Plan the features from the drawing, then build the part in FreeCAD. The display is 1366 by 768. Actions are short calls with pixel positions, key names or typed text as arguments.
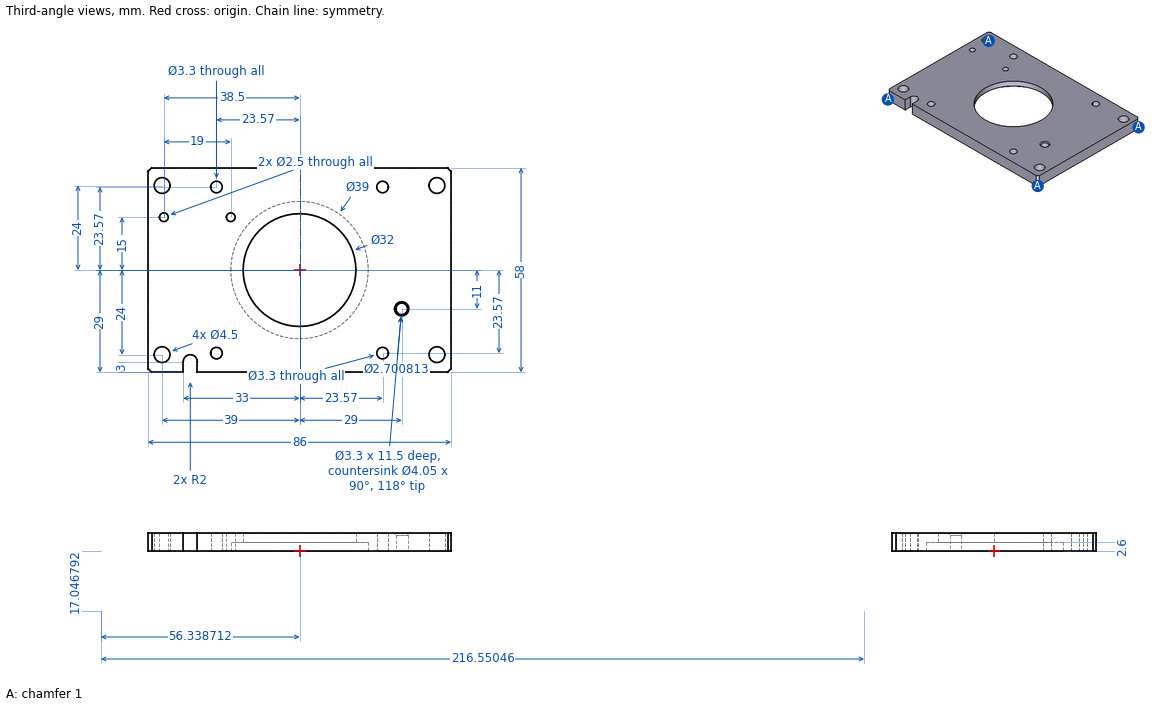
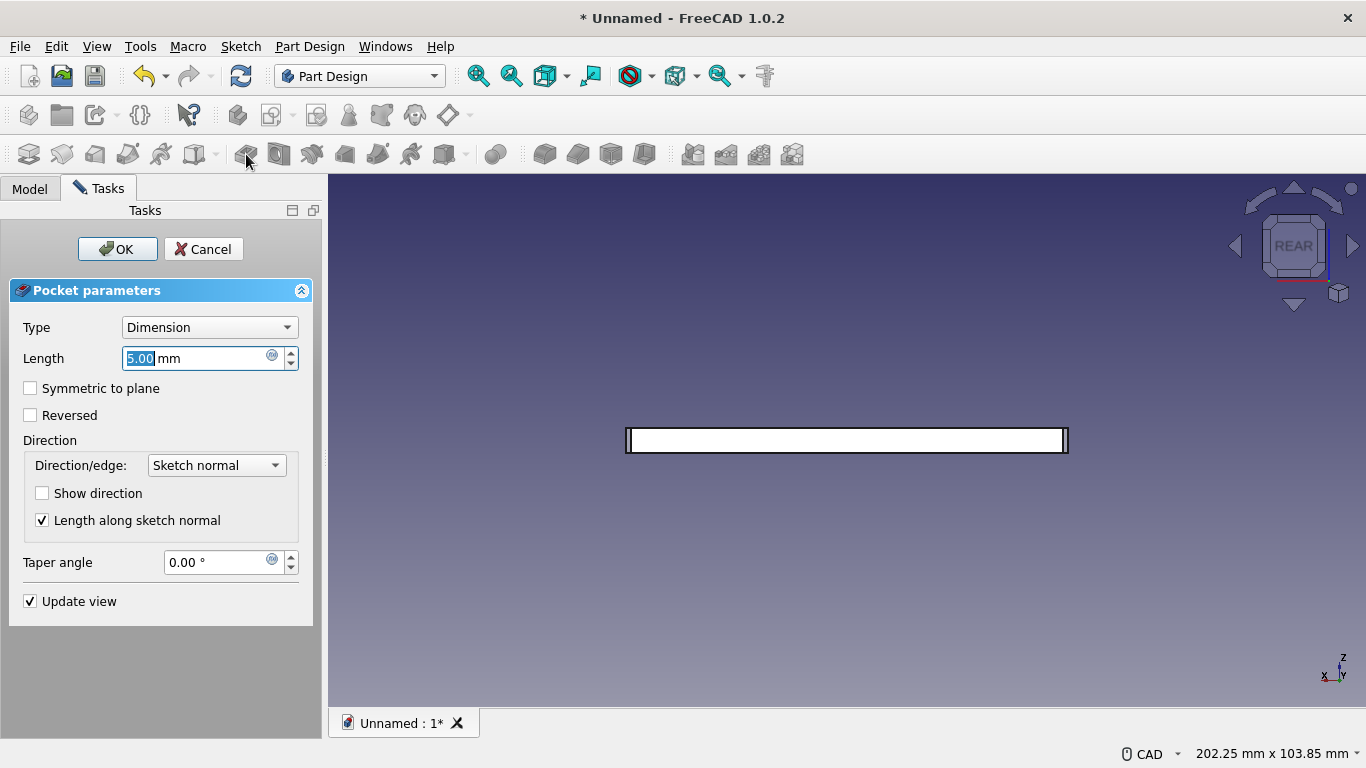
text(2.6)
key(Tab)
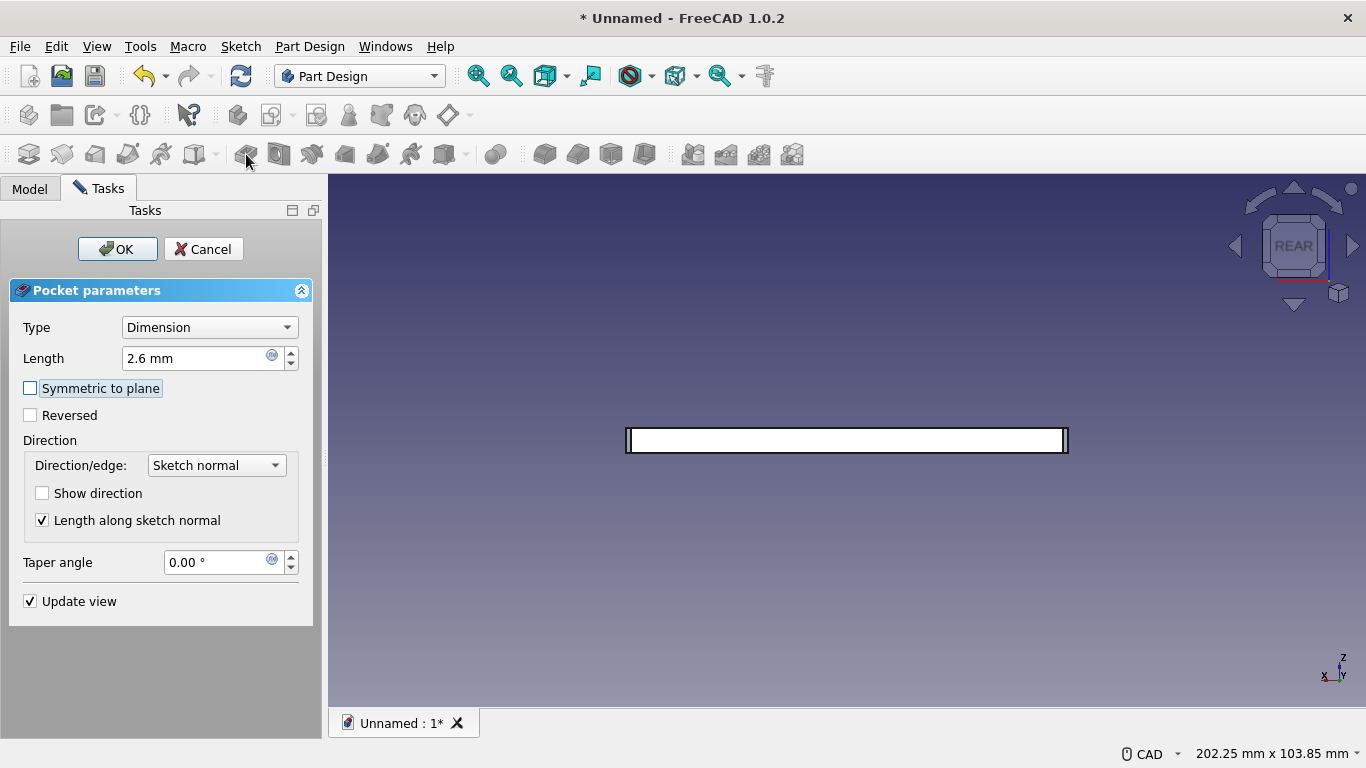
click(31, 415)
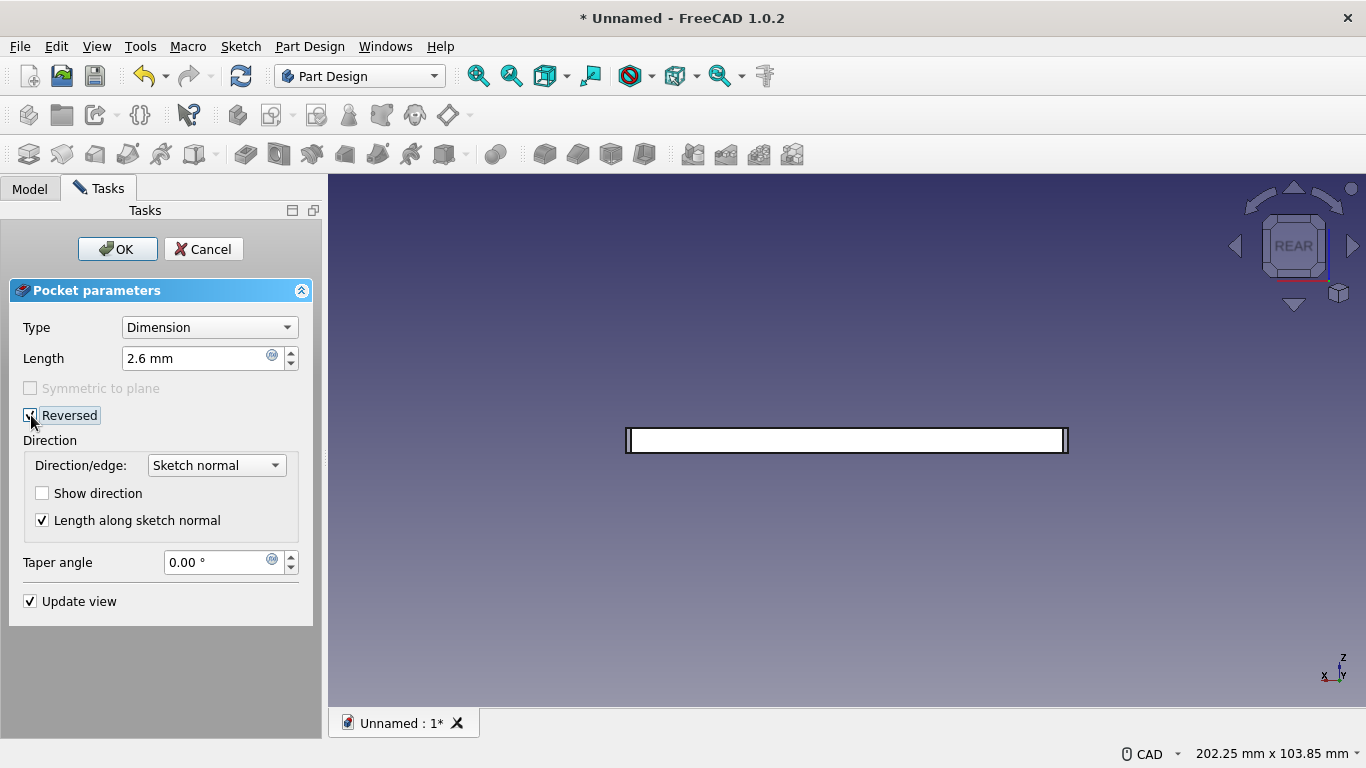
click(118, 249)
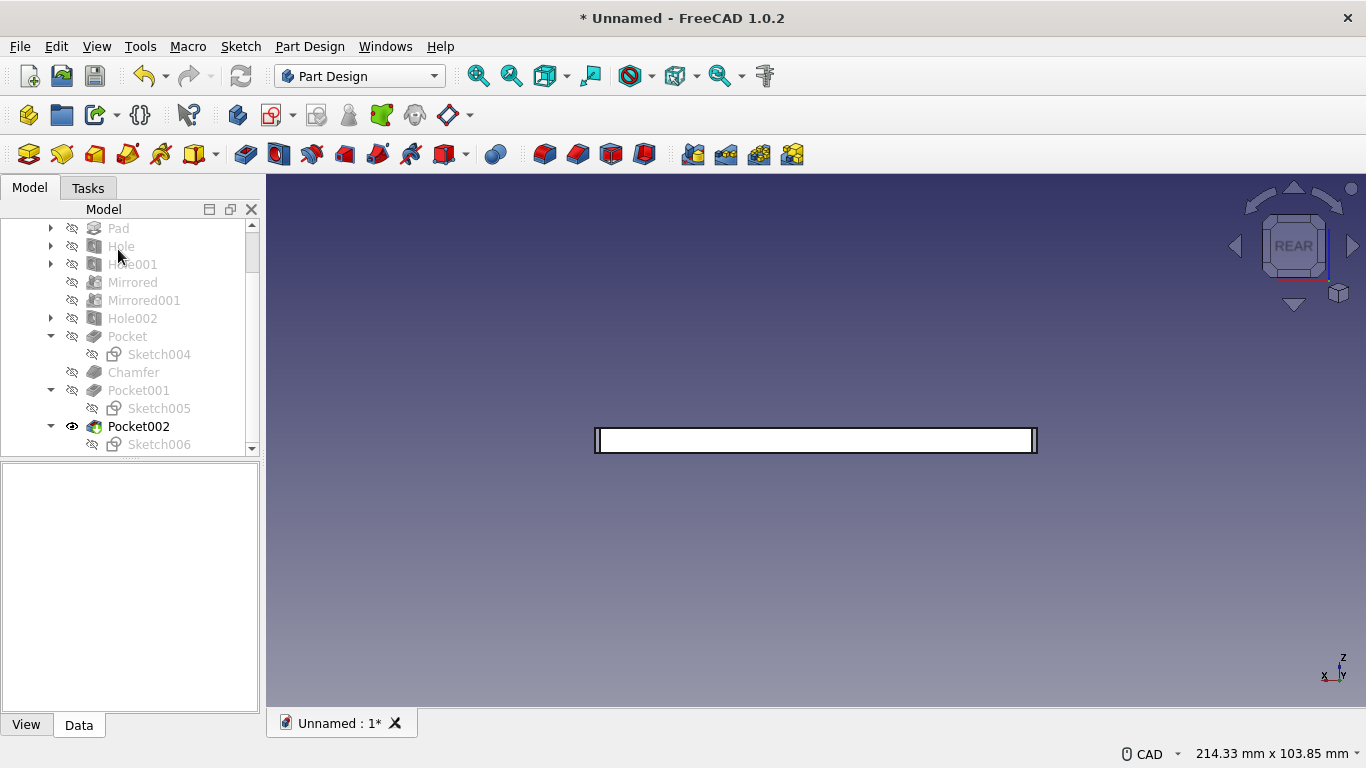
click(479, 76)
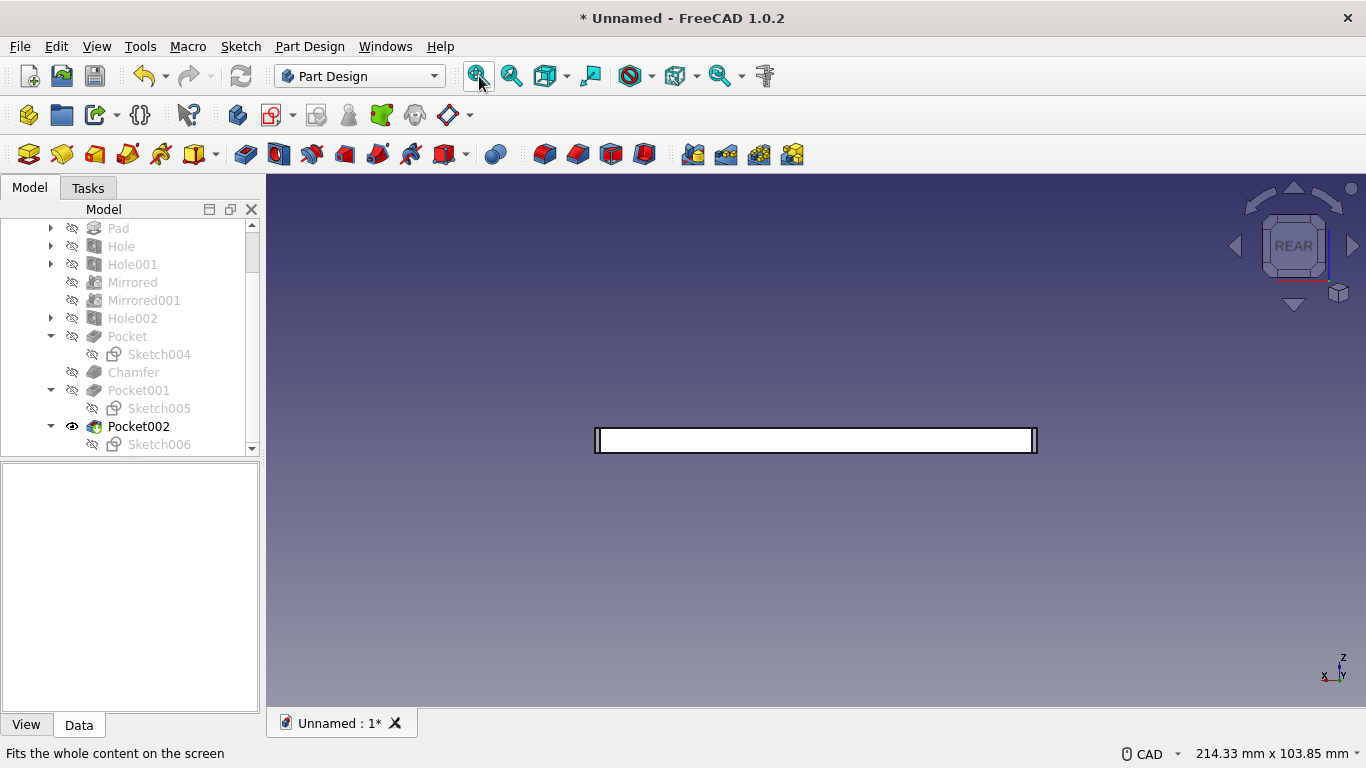
key(0)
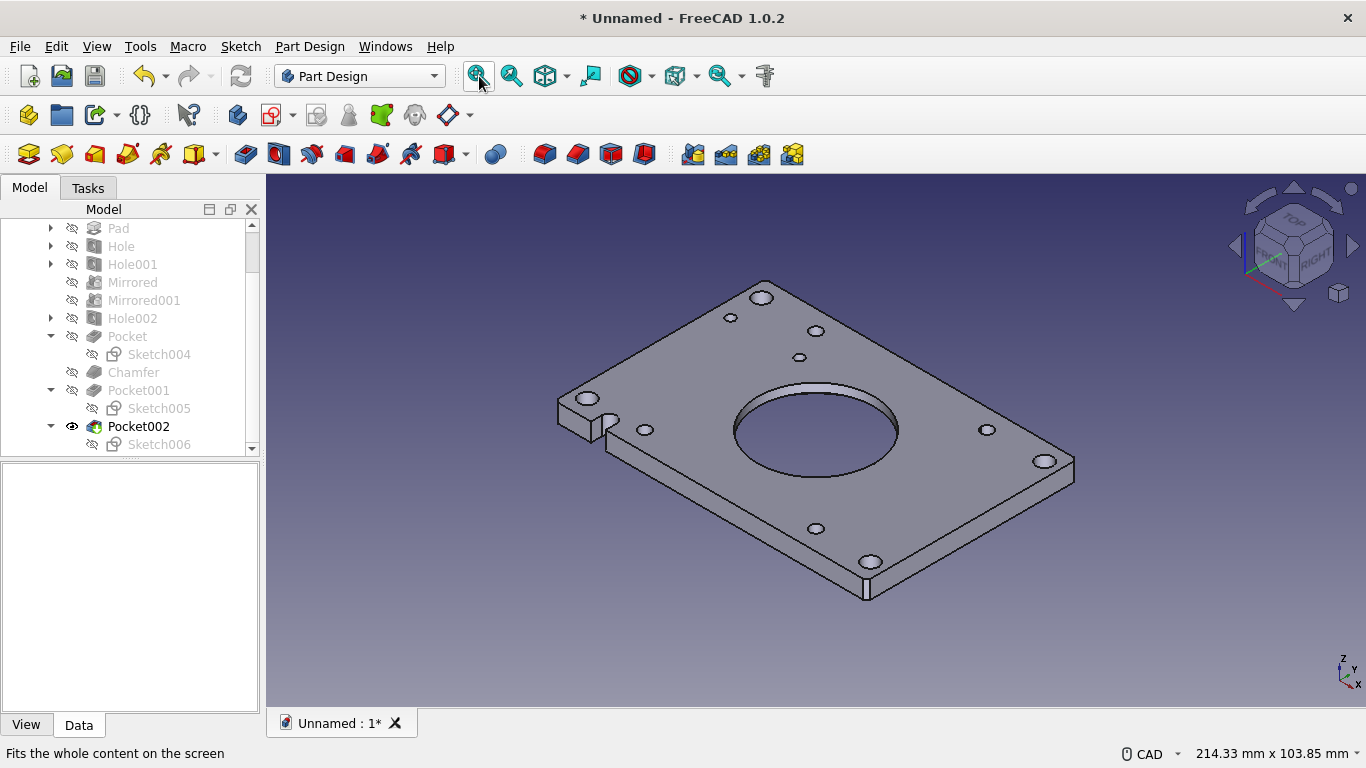
click(697, 395)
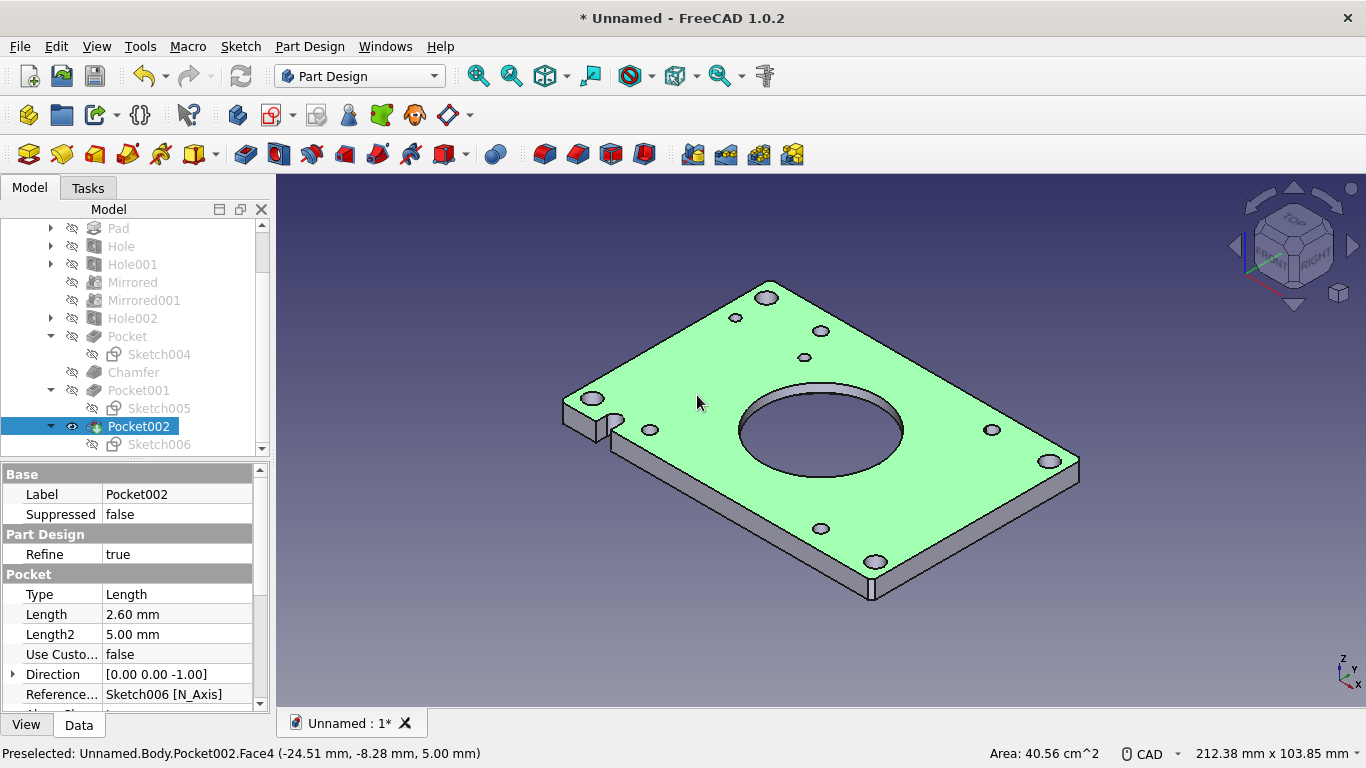
click(270, 116)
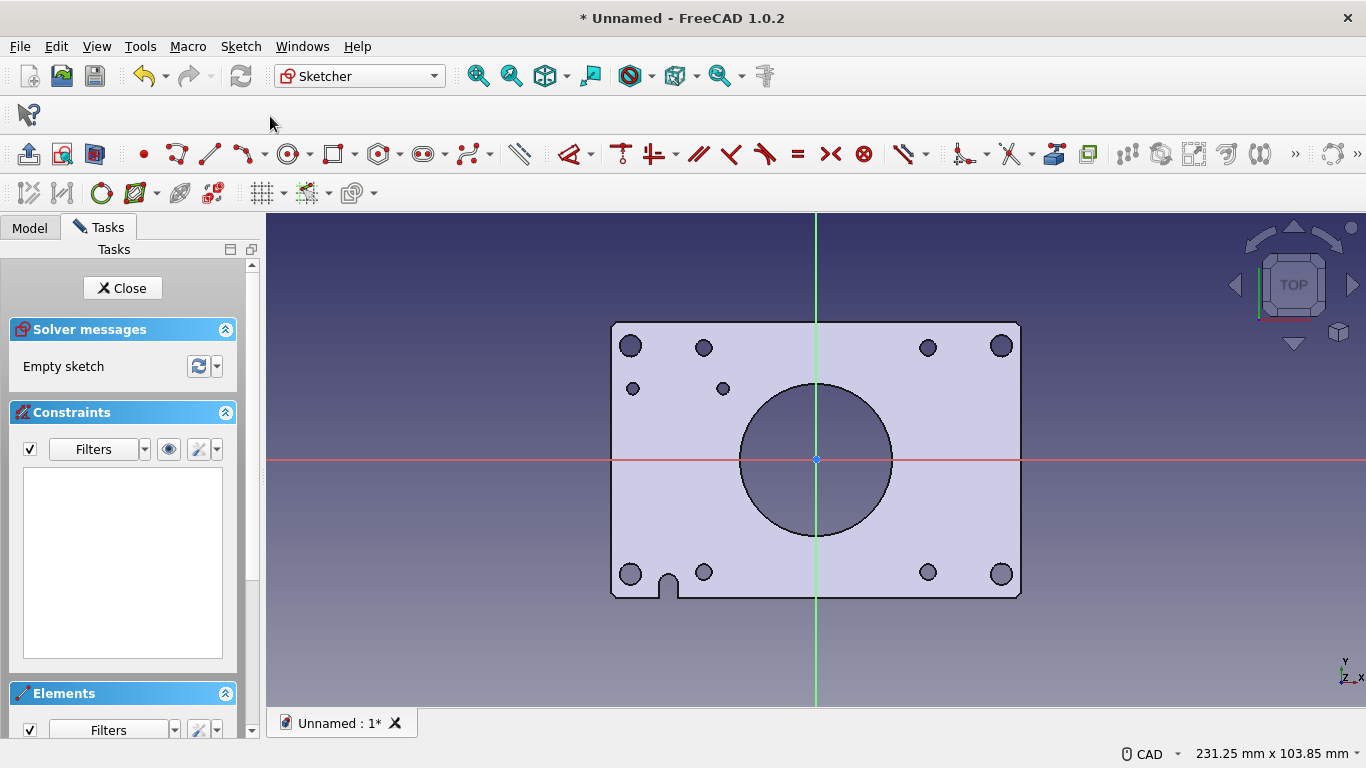
scroll(965, 515, up, 15)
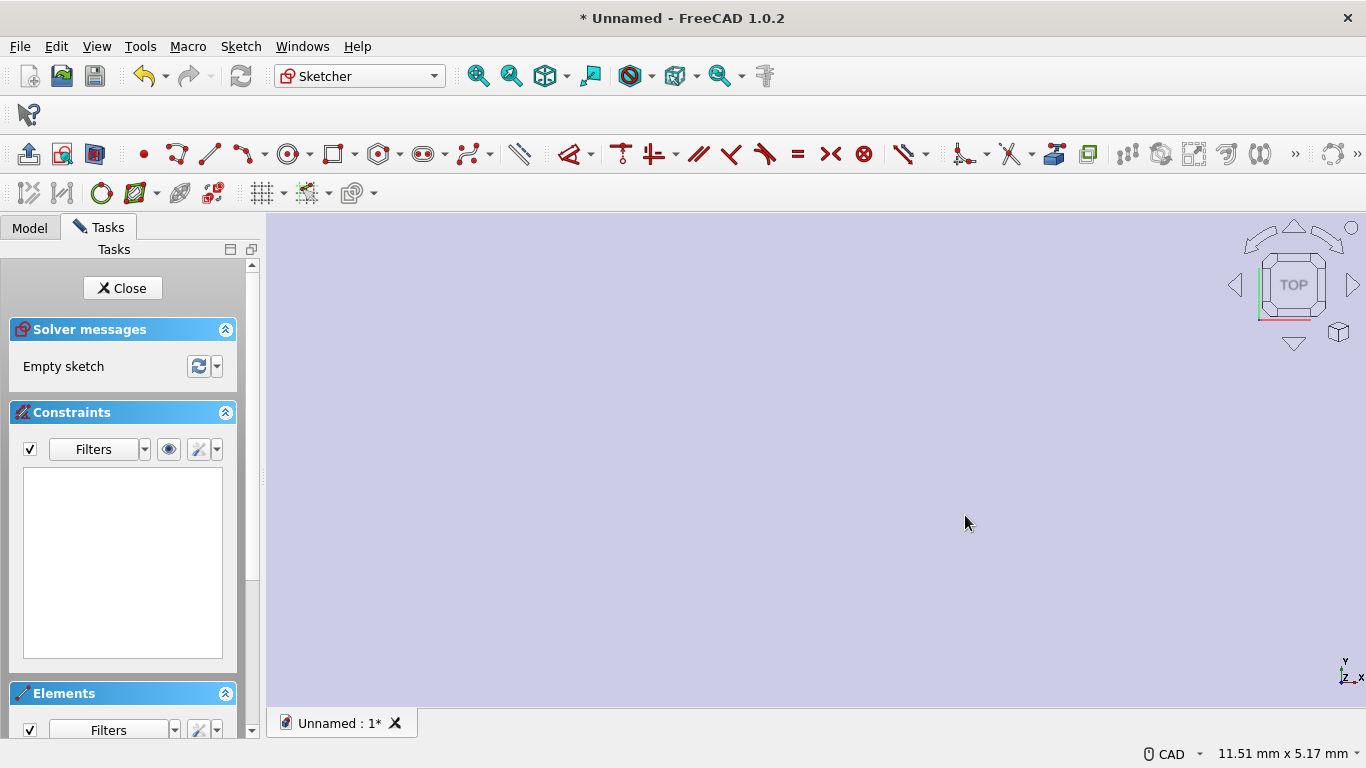
click(288, 154)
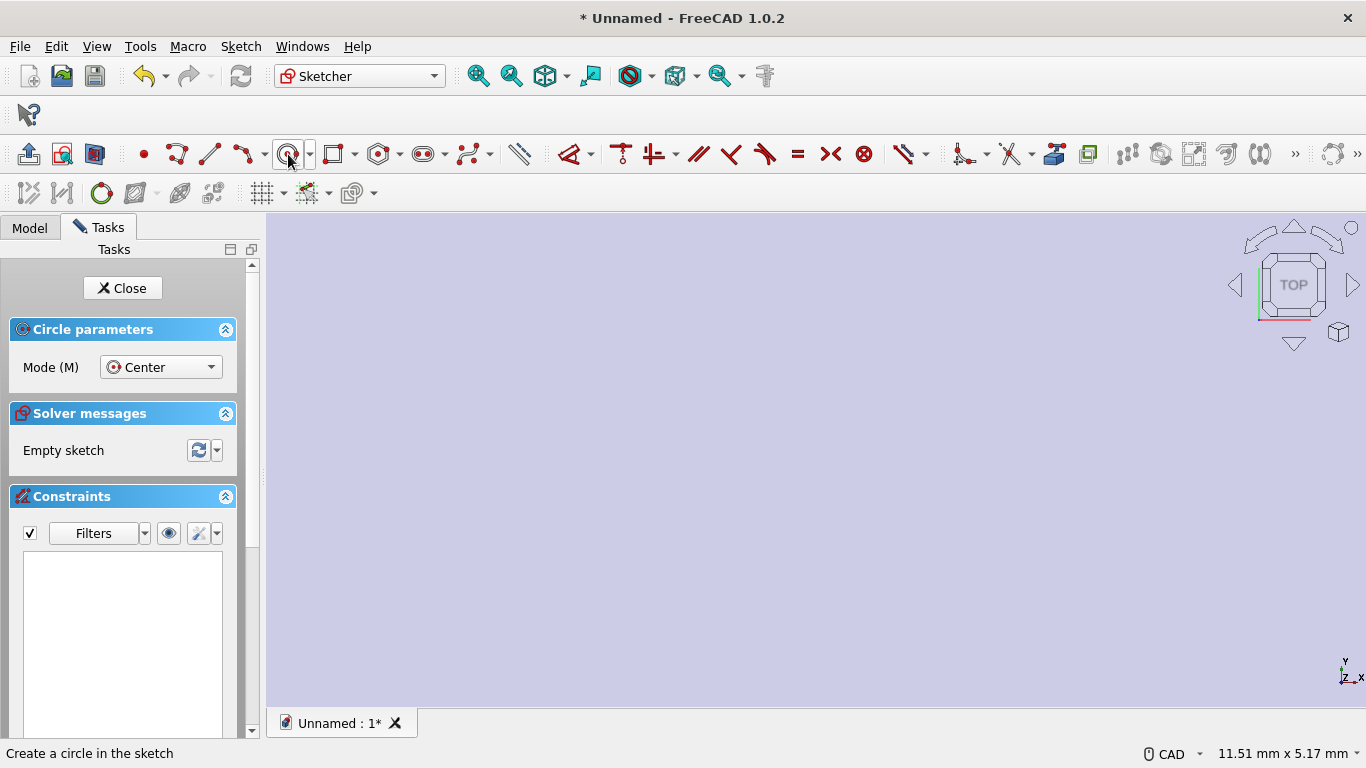
click(731, 450)
move(822, 358)